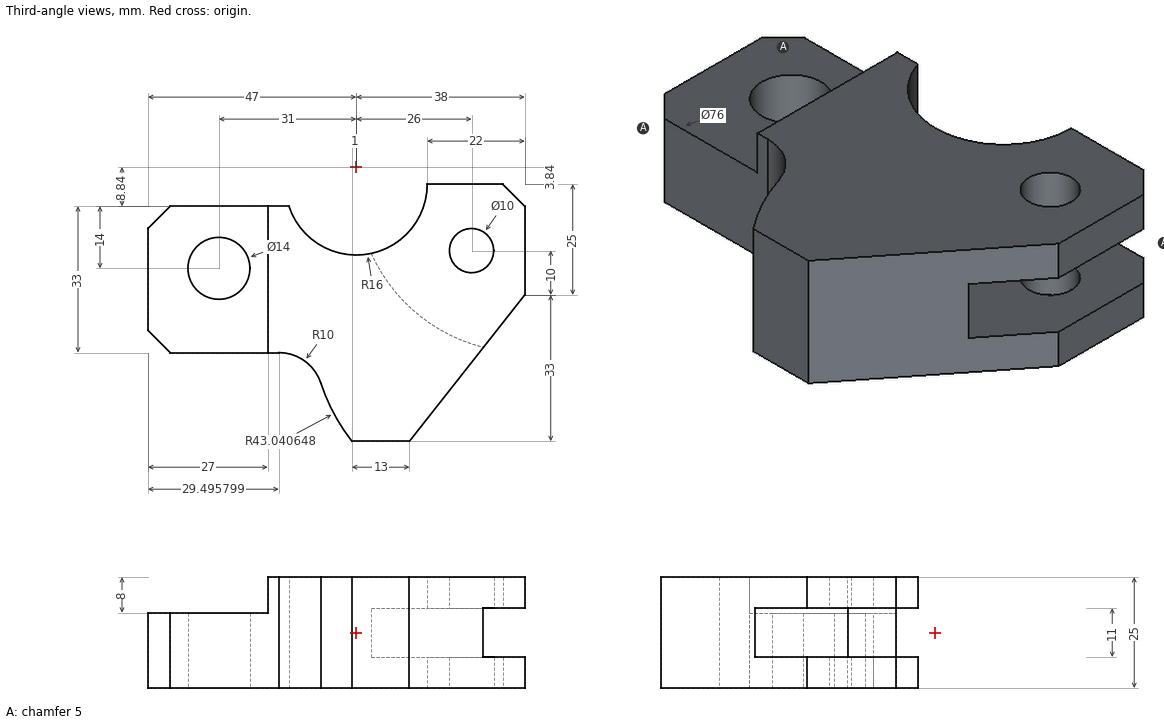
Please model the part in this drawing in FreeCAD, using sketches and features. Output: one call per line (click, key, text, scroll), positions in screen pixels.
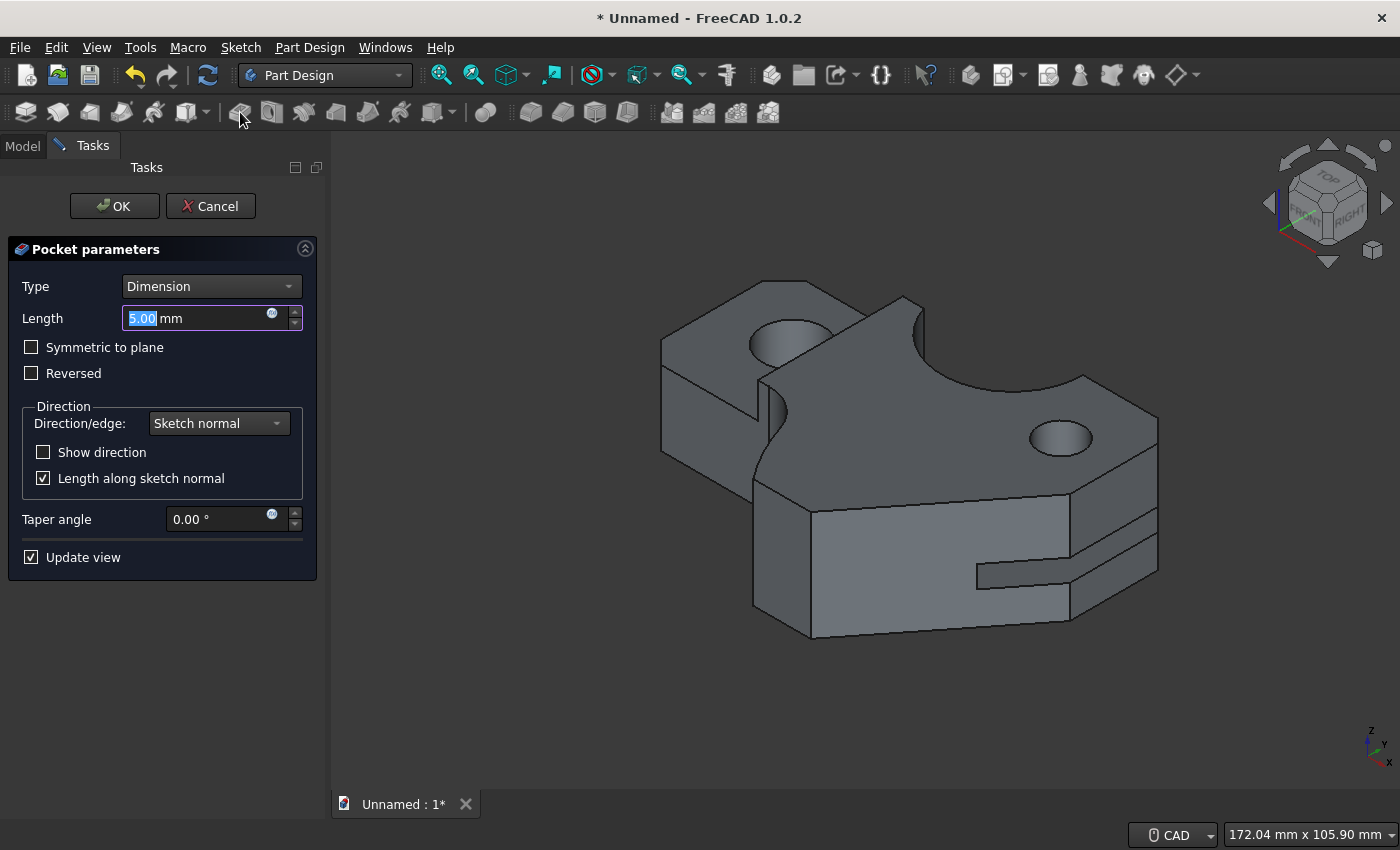
text(11)
key(Tab)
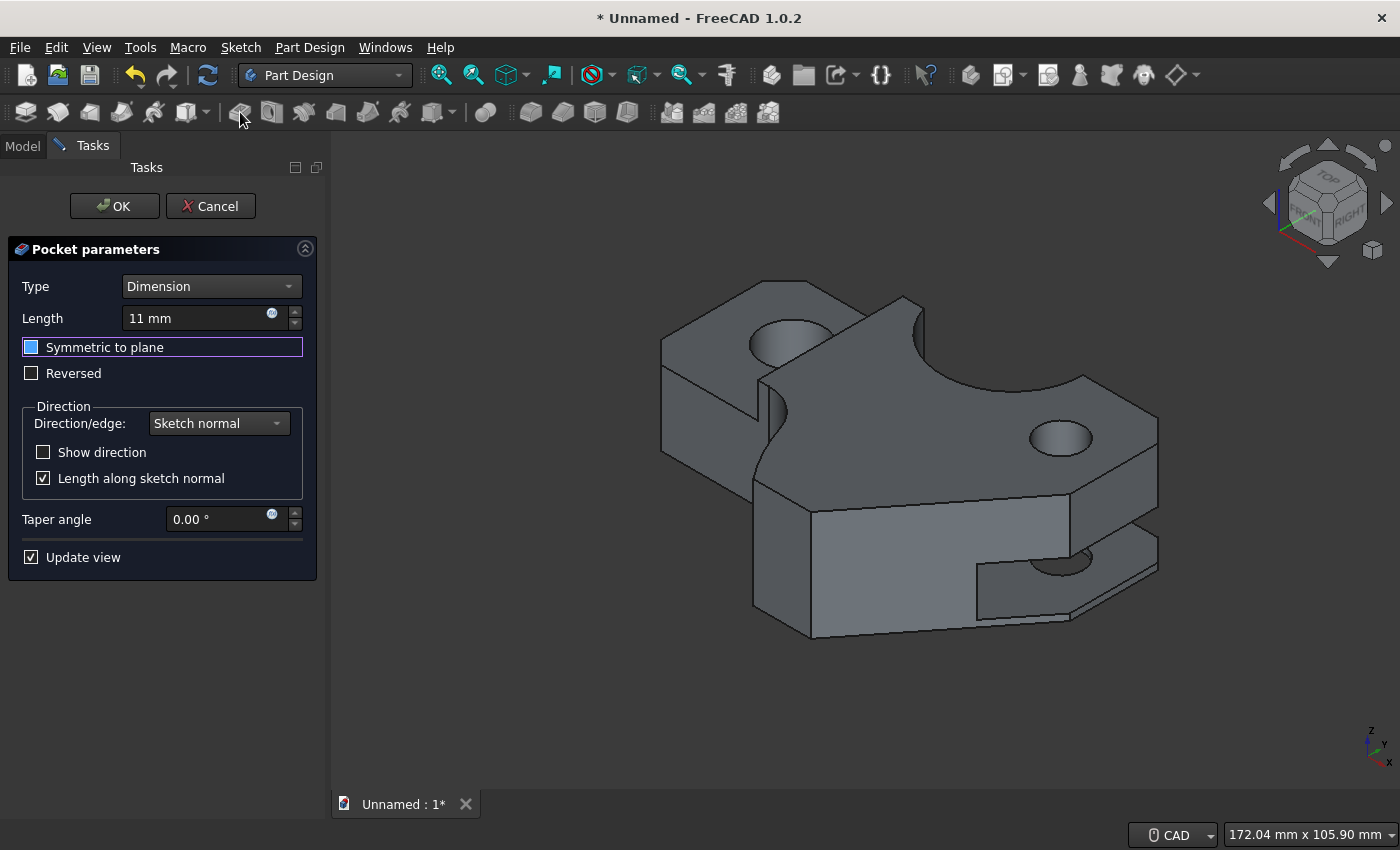
click(30, 347)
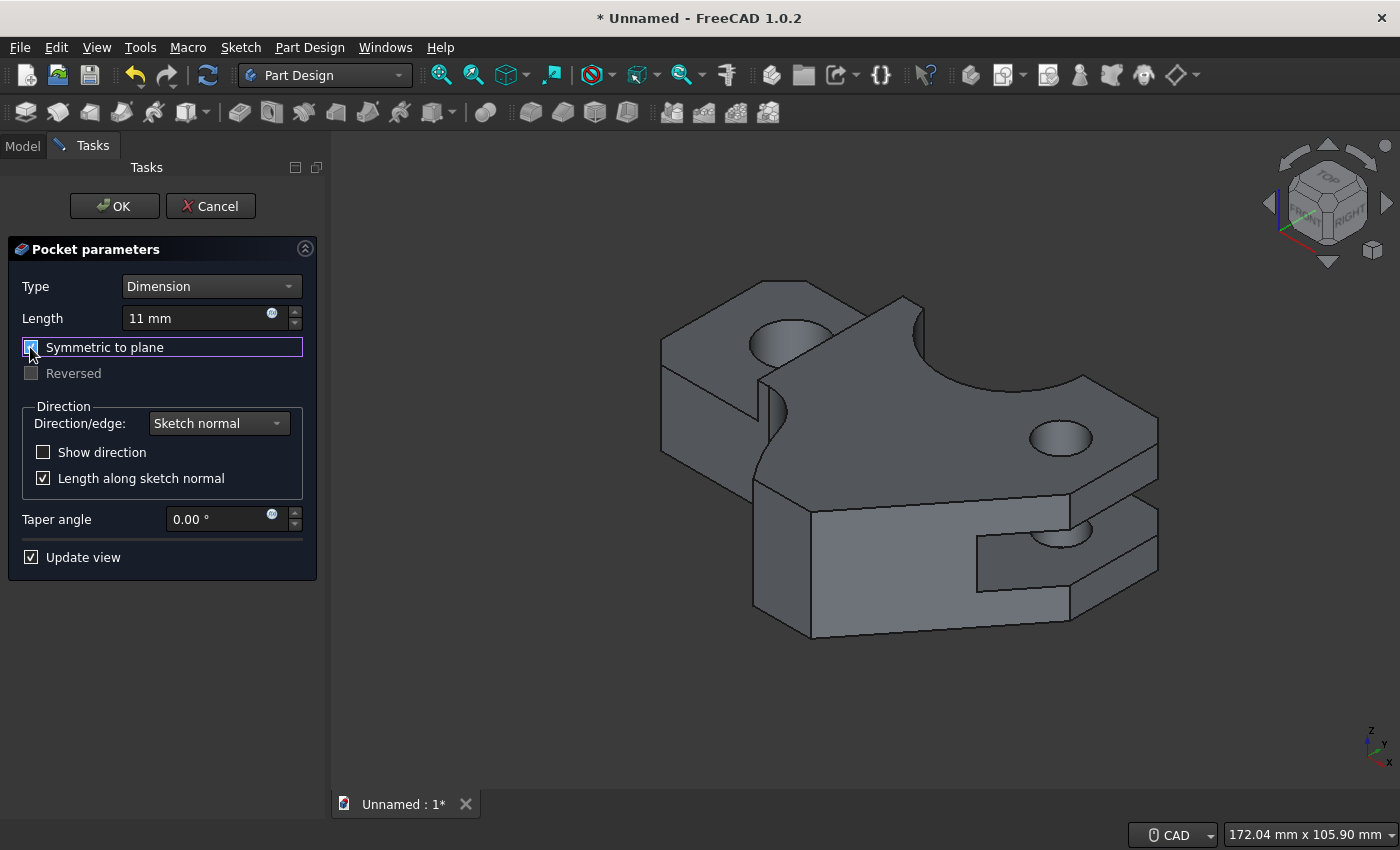
click(115, 206)